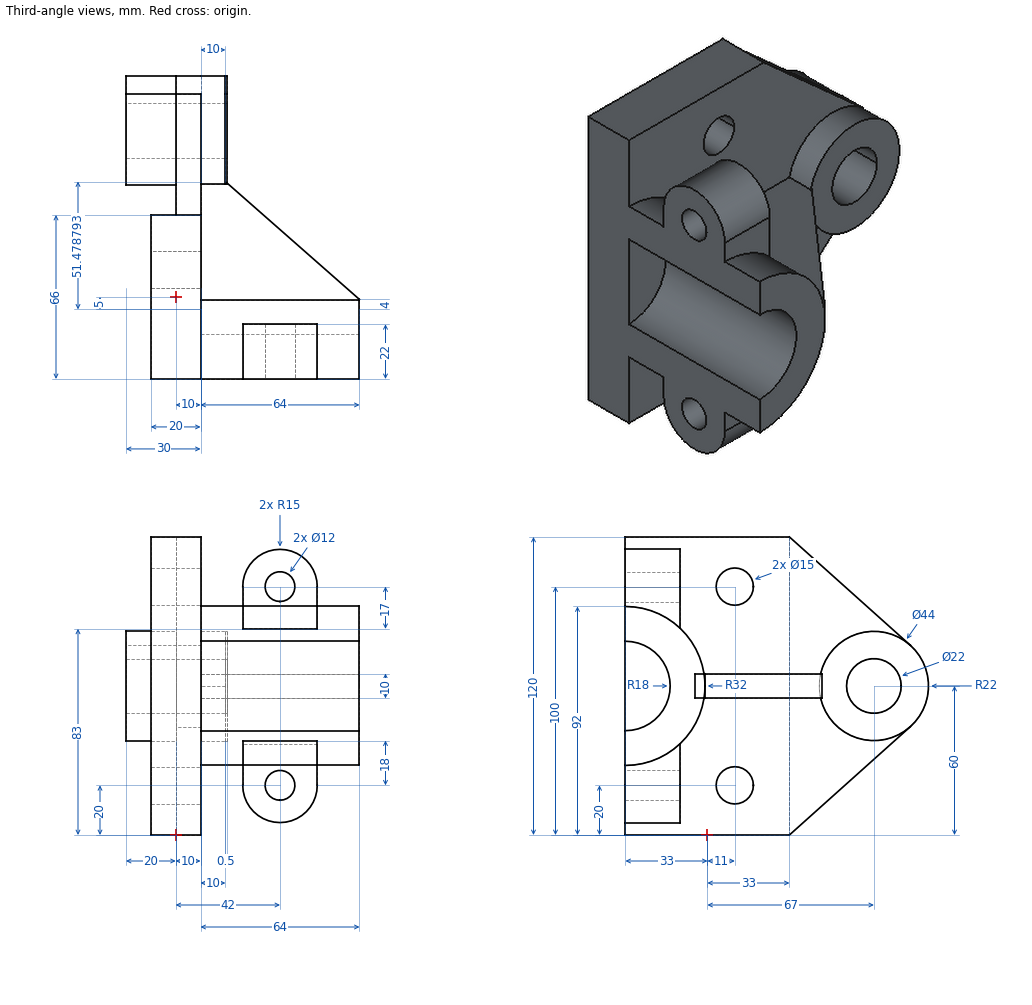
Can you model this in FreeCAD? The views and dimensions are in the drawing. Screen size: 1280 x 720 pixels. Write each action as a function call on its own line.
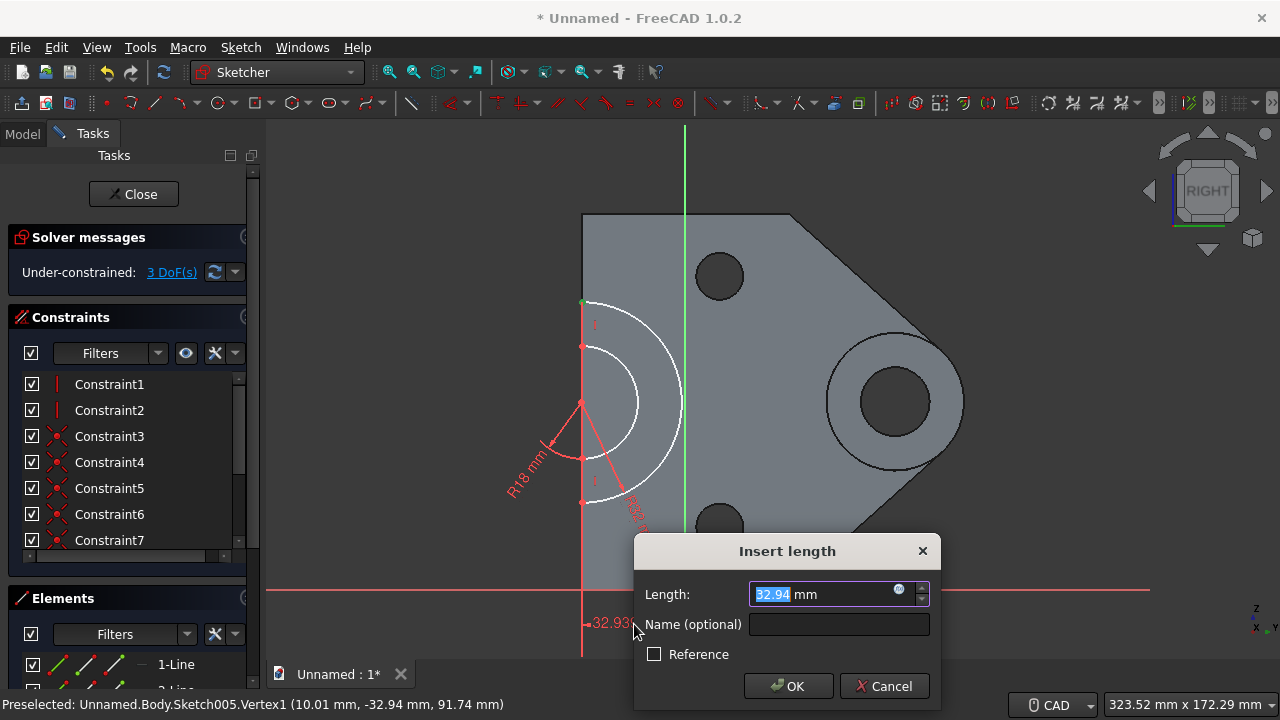
text(33)
key(Return)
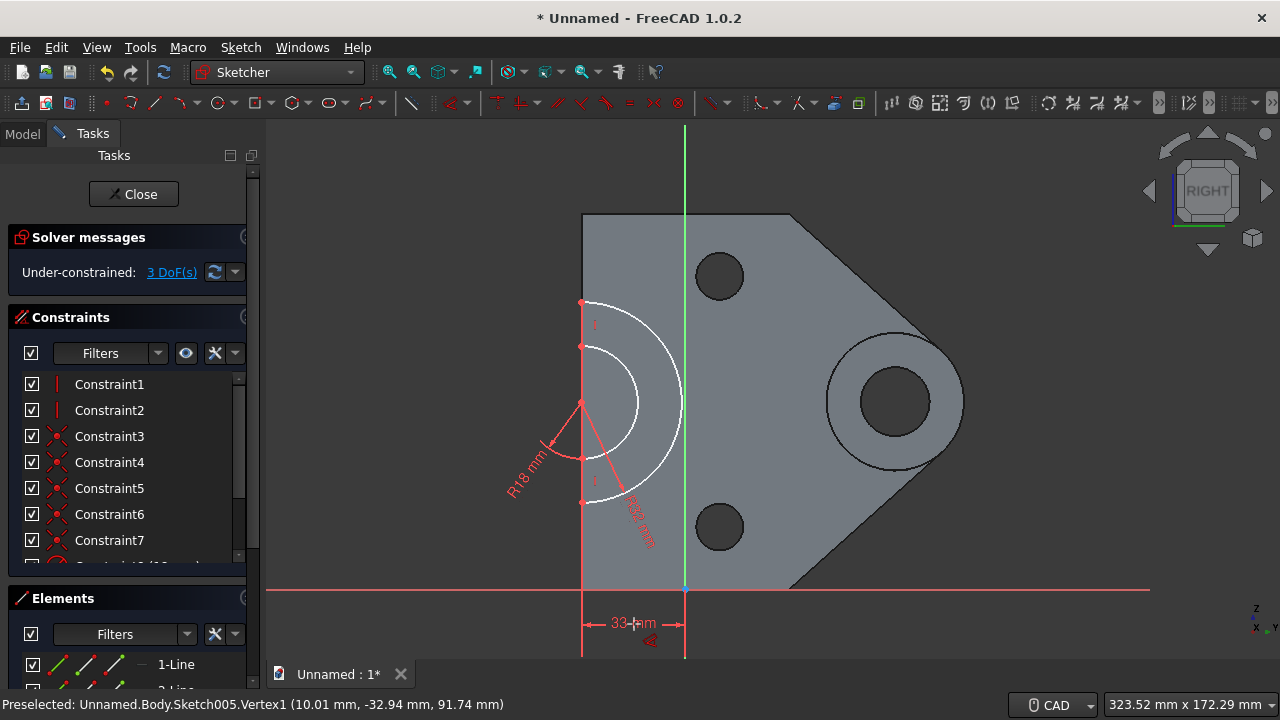
click(582, 302)
click(719, 446)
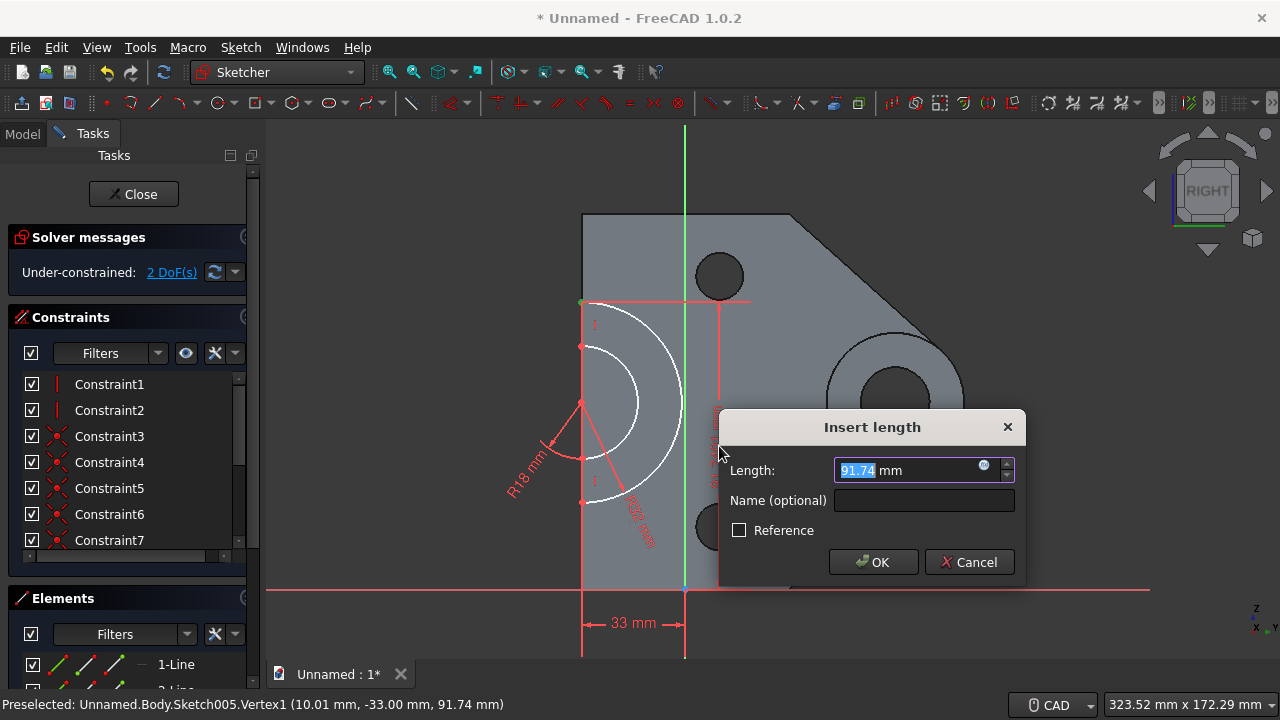
text(92)
key(Return)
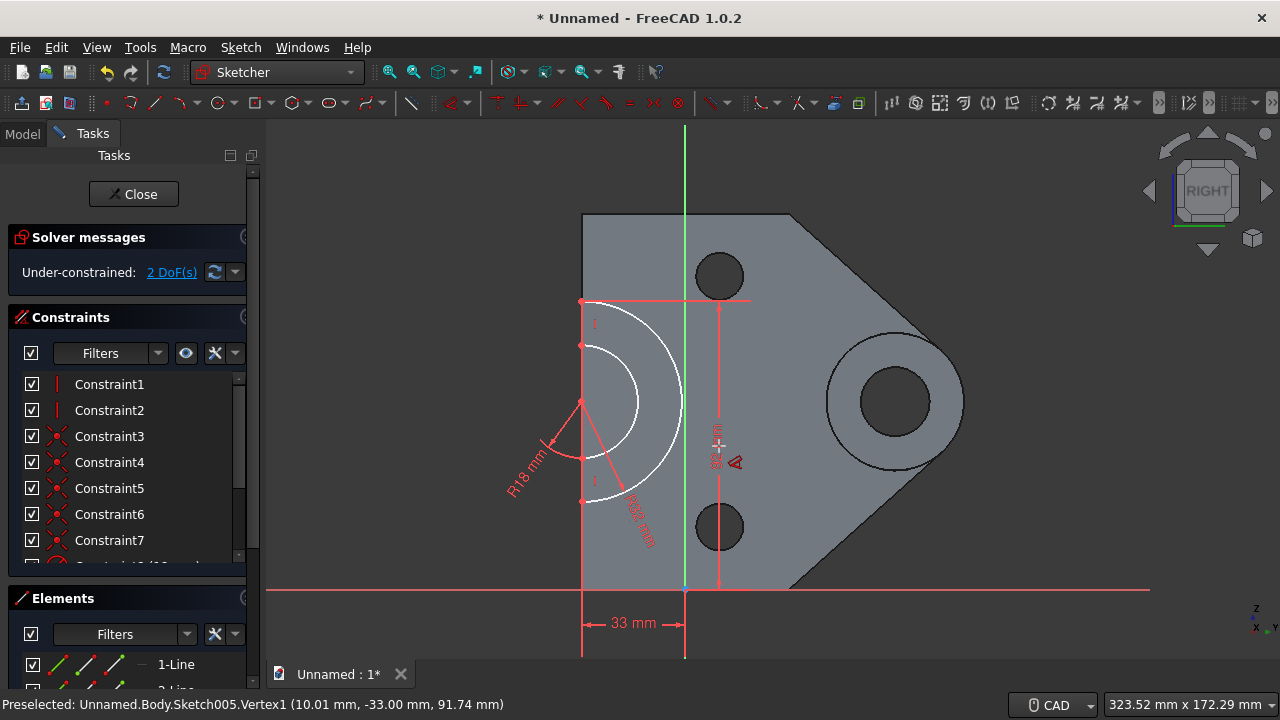
click(582, 458)
click(610, 424)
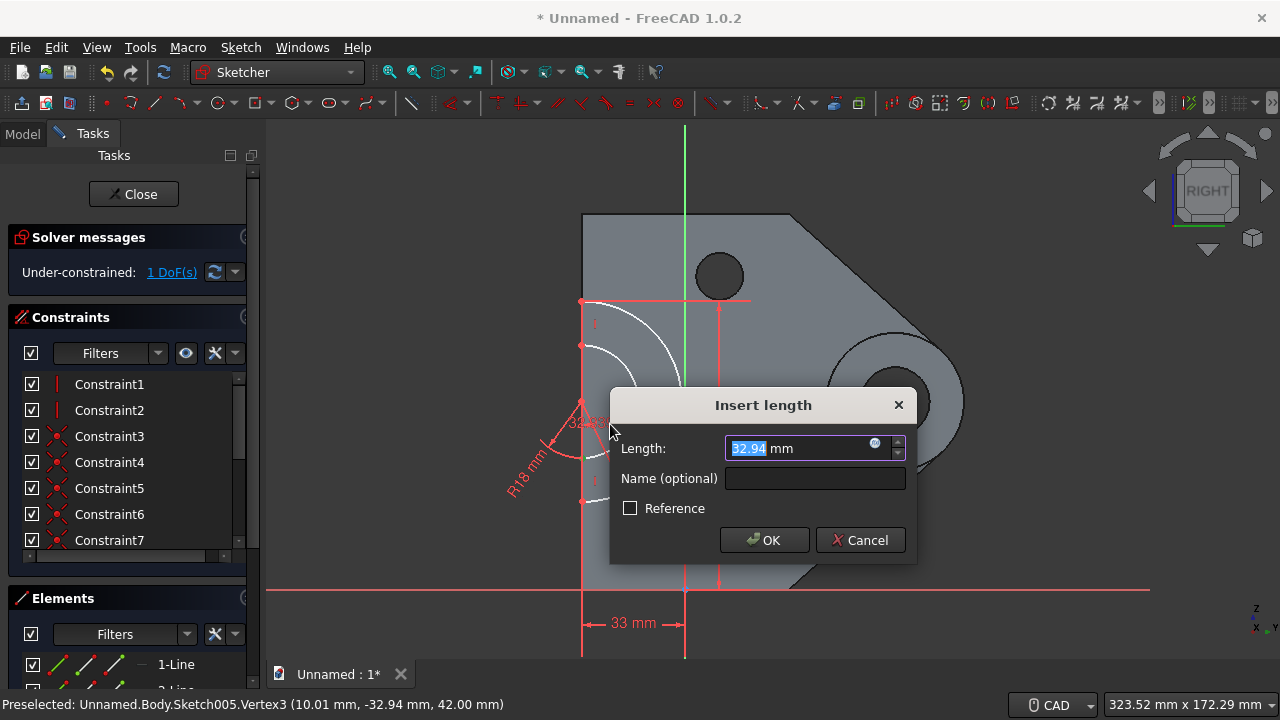
text(33)
key(Return)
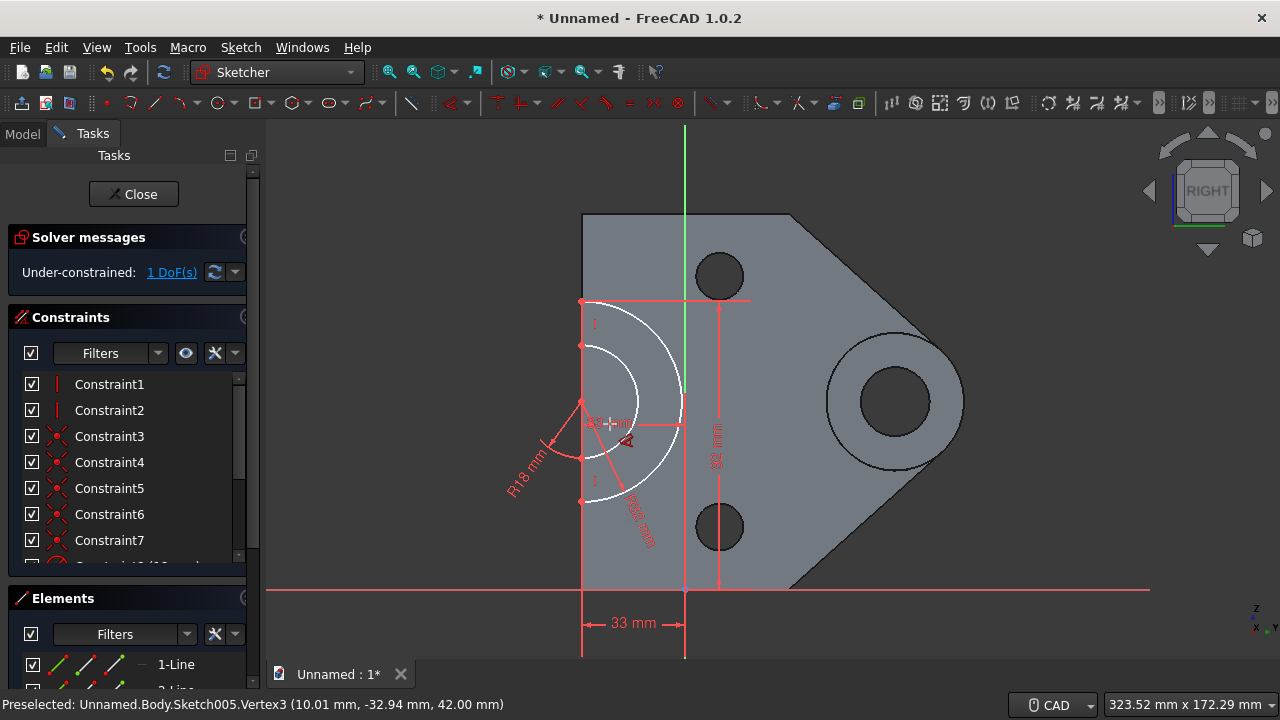
click(582, 402)
click(657, 368)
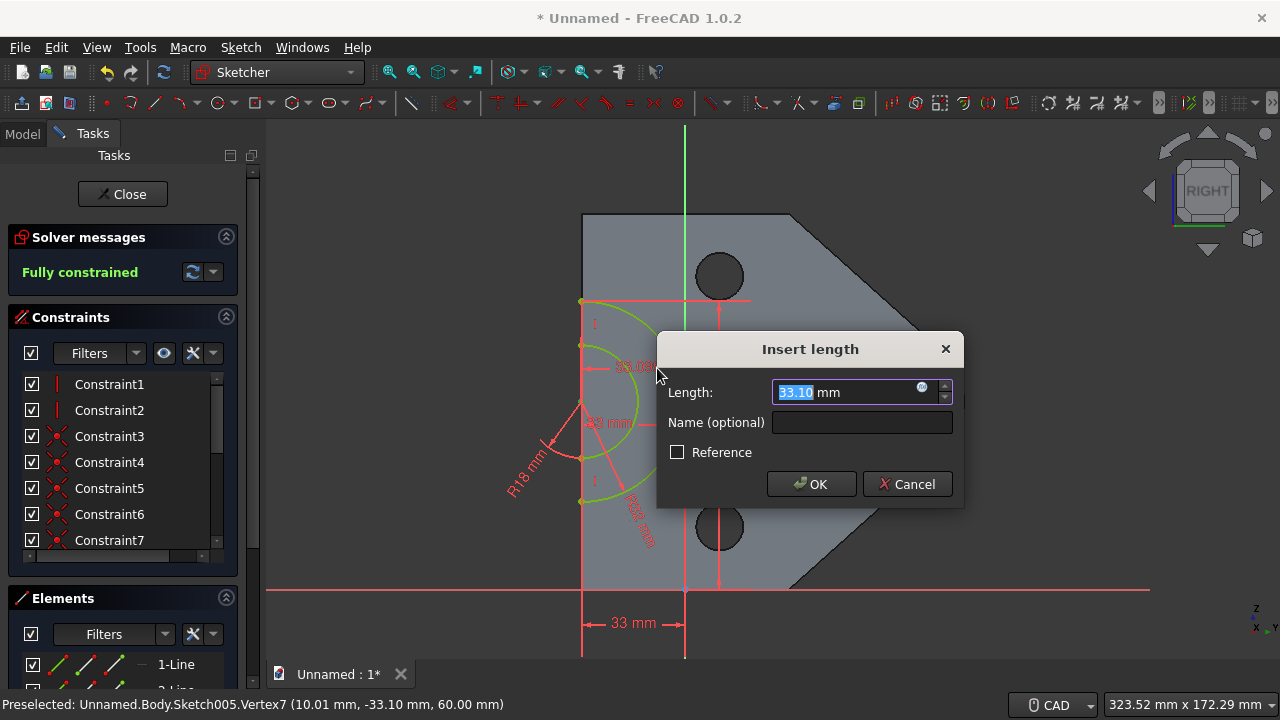
text(33)
key(Return)
key(Escape)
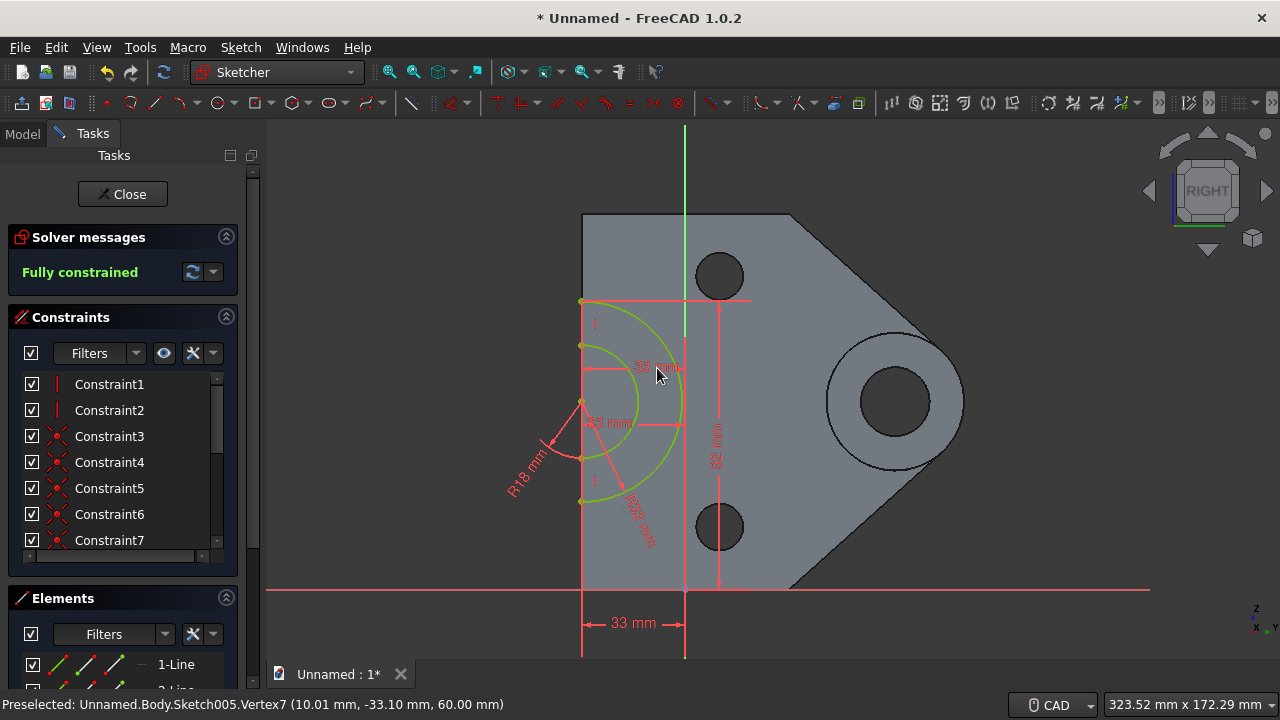
click(123, 194)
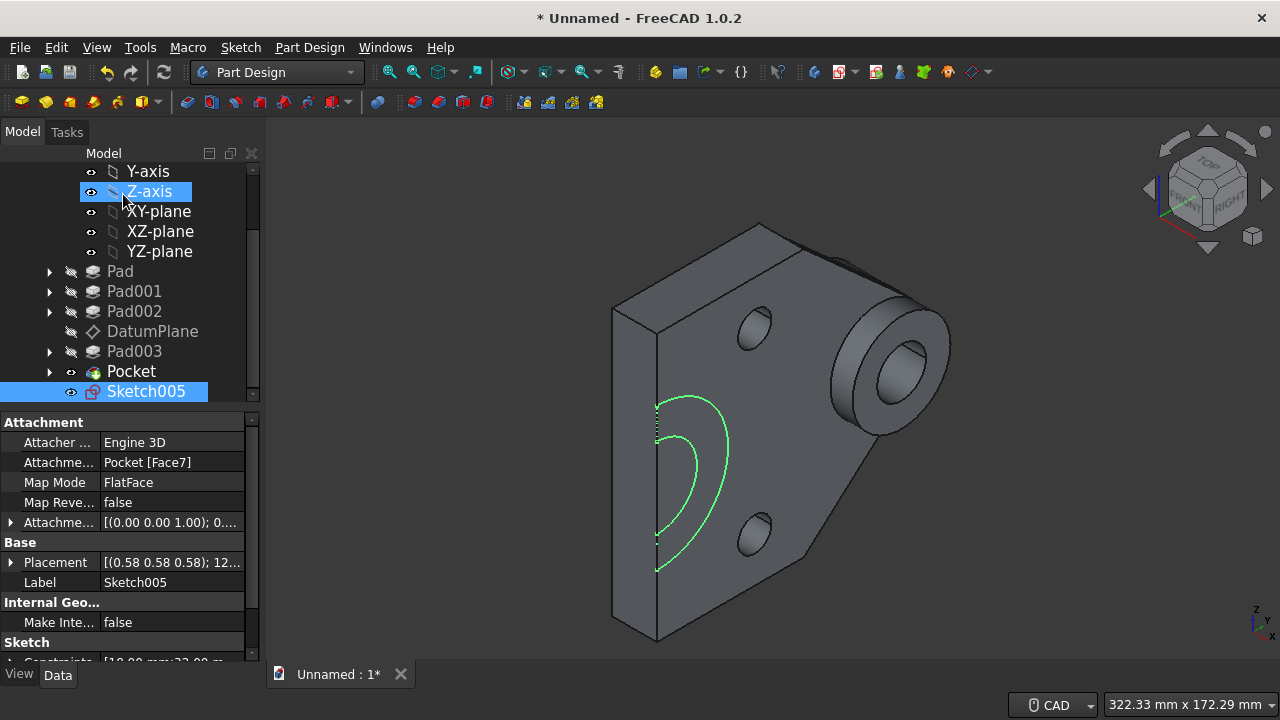
click(22, 102)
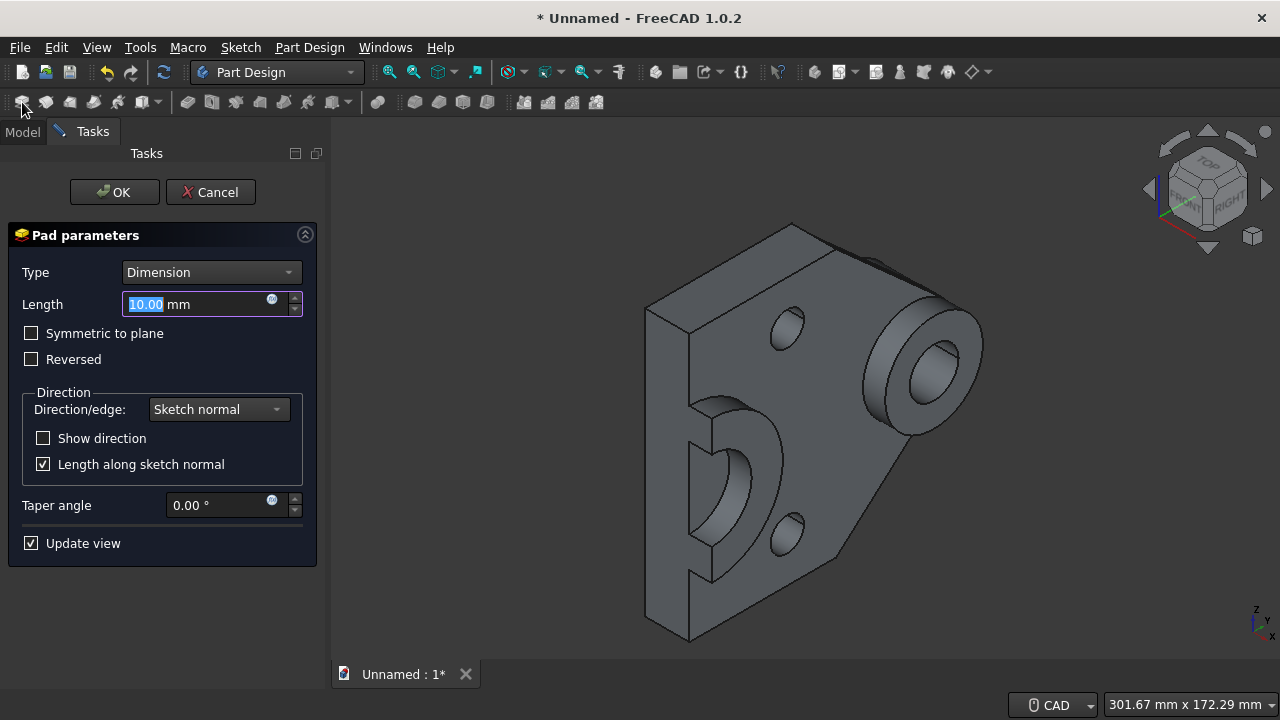
text(64)
key(Tab)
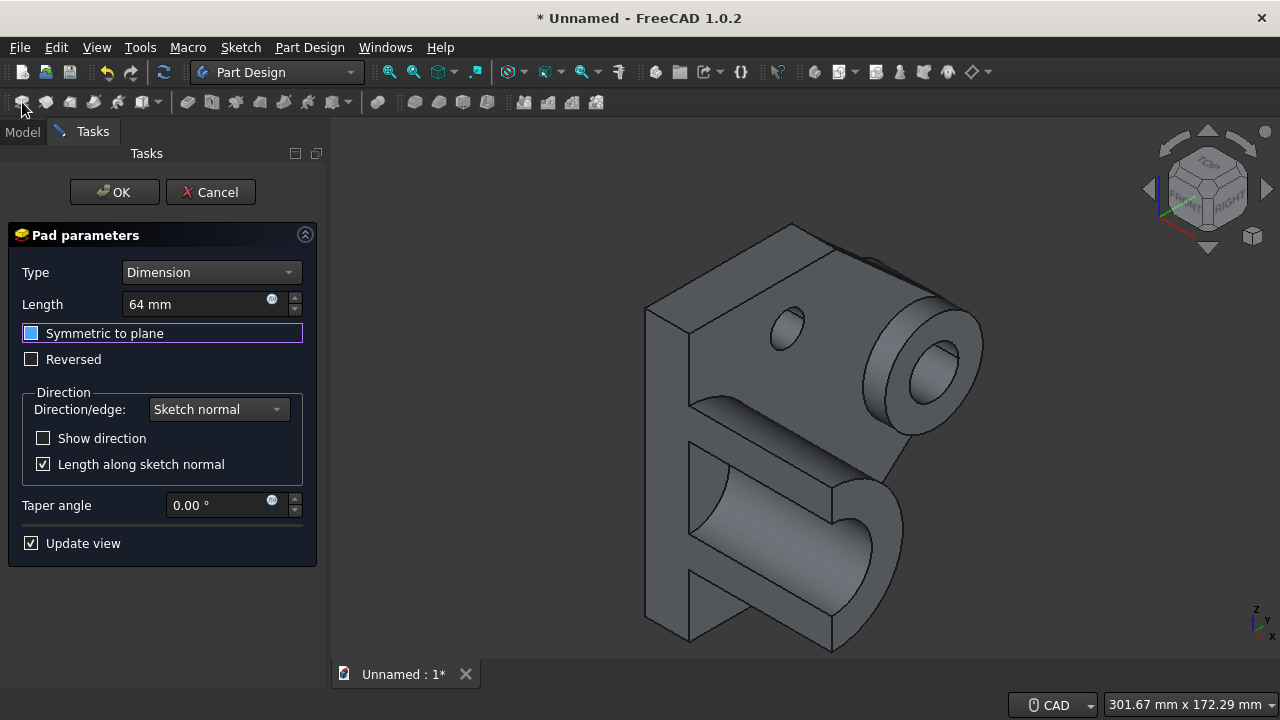
click(115, 192)